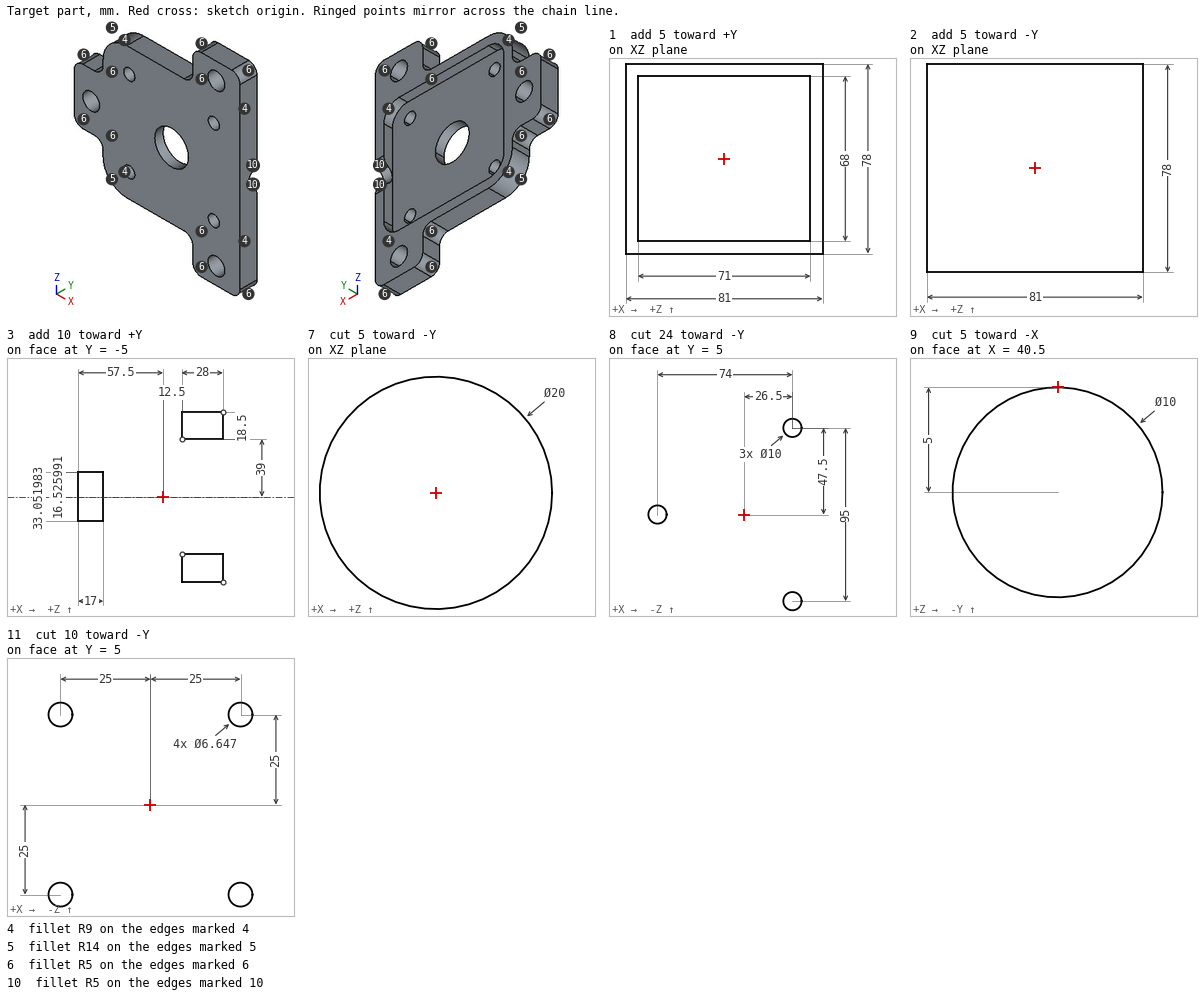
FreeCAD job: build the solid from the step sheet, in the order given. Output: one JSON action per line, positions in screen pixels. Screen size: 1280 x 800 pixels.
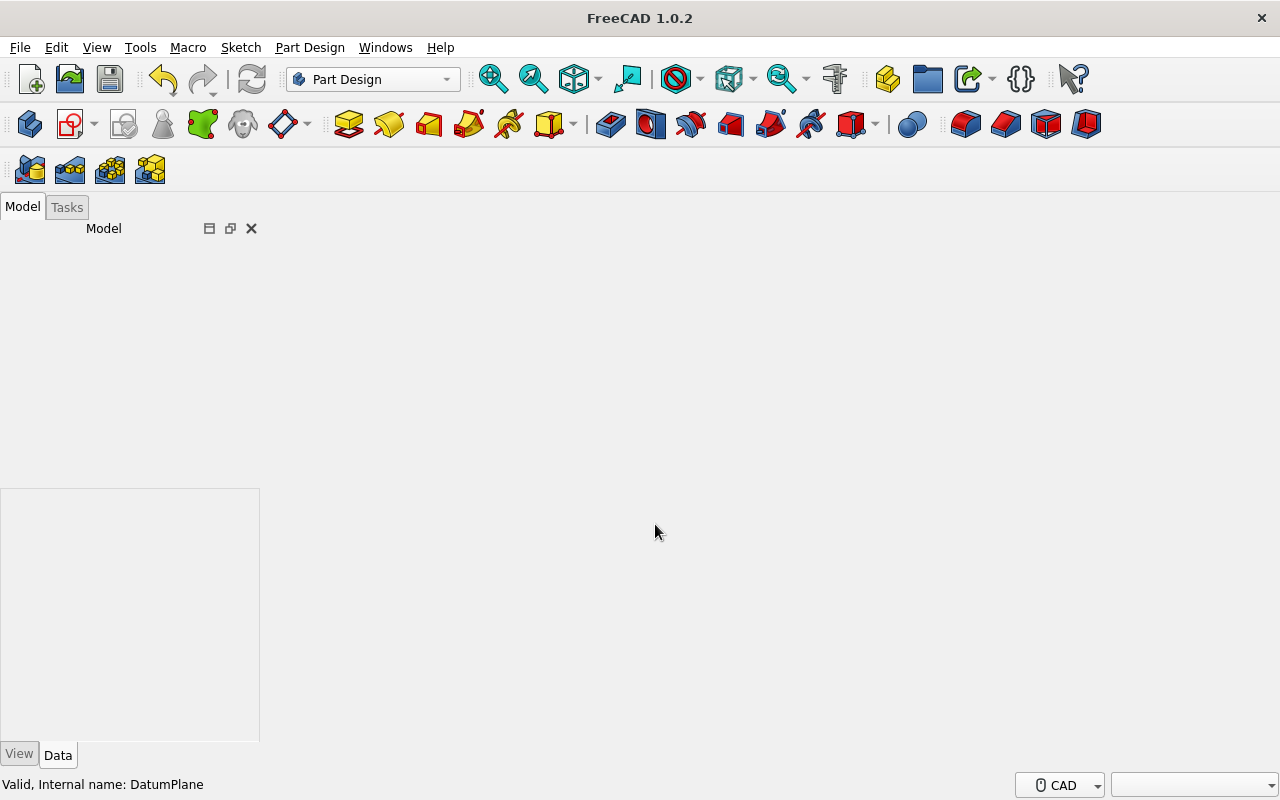
{"action": "left_click", "coordinate": [30, 80]}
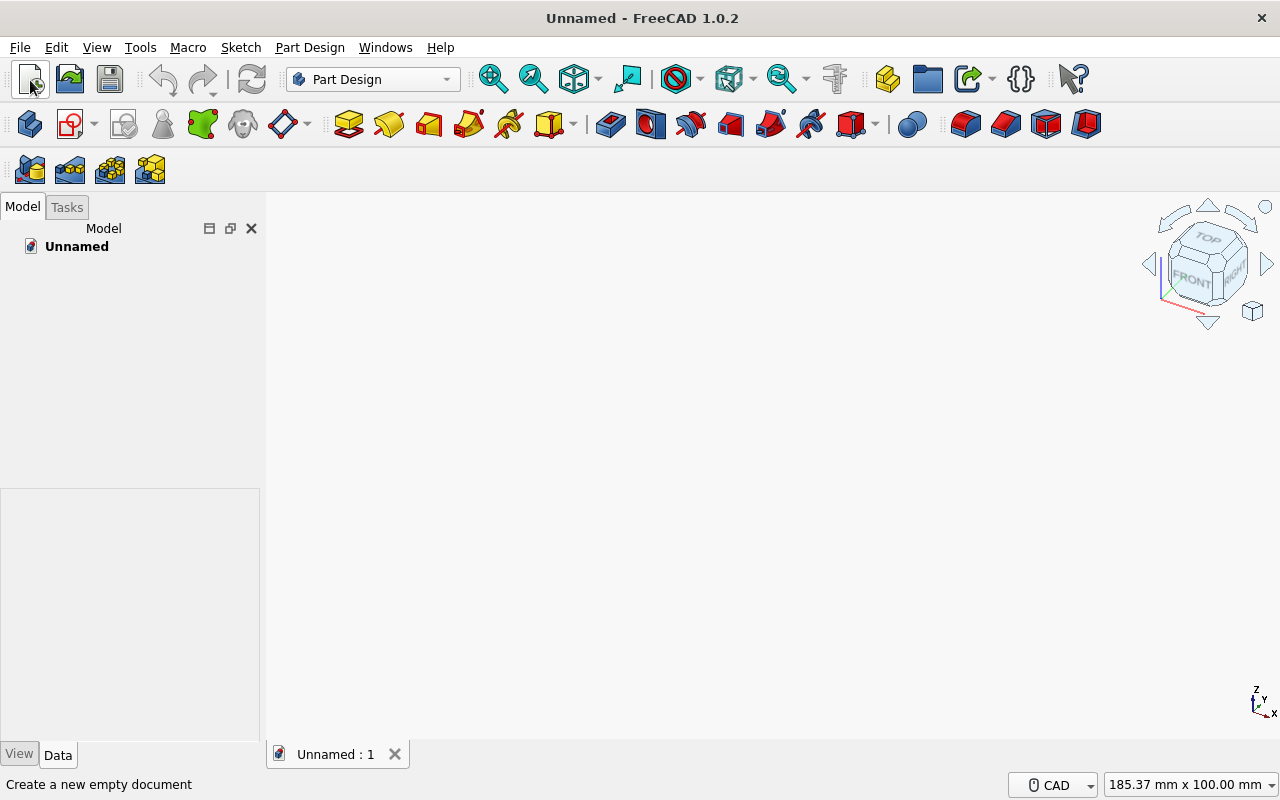
{"action": "left_click", "coordinate": [70, 124]}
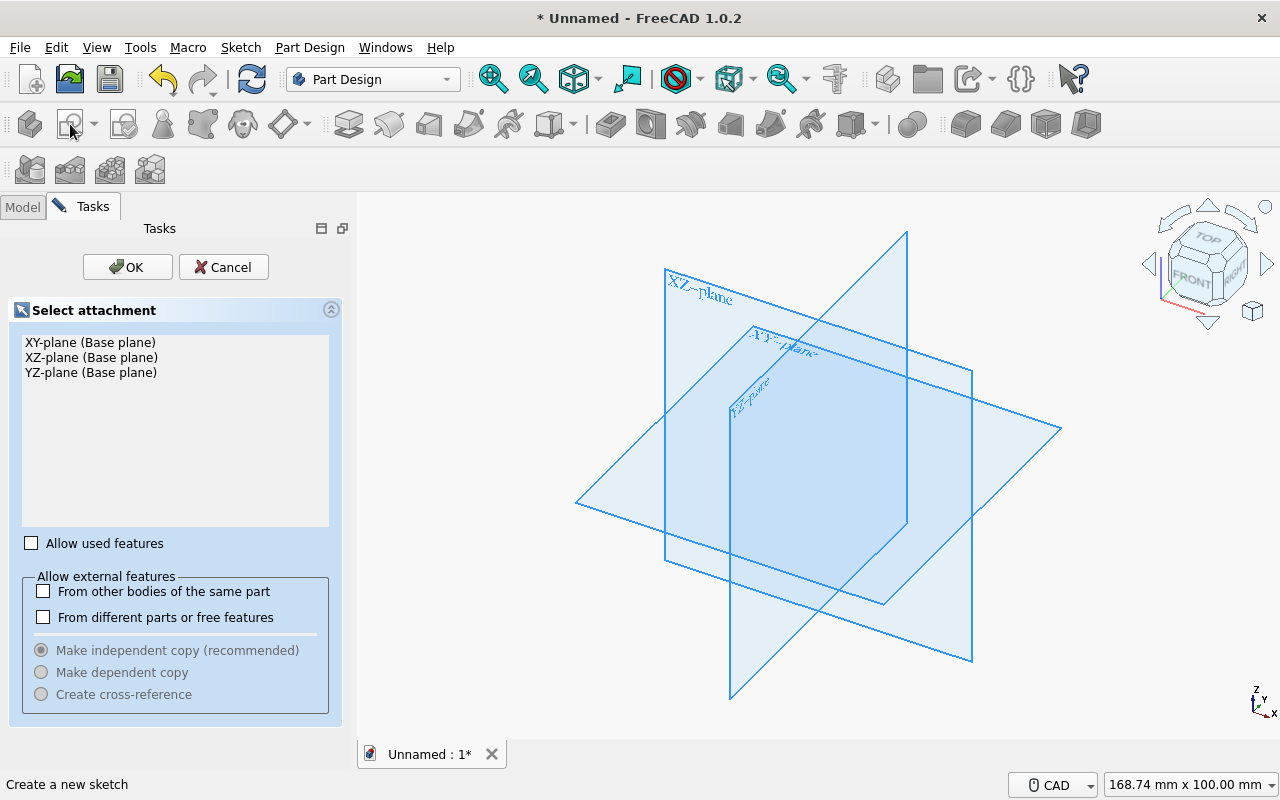
{"action": "left_click", "coordinate": [82, 358]}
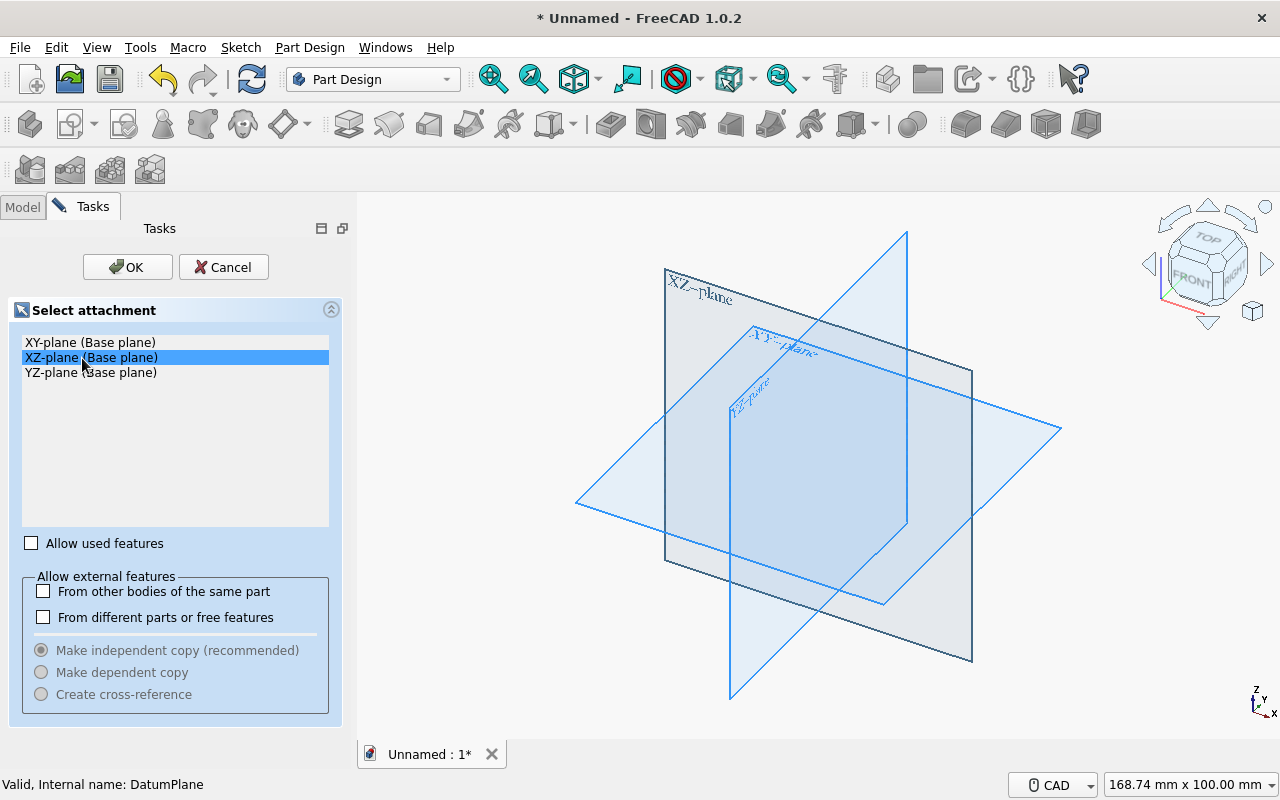
{"action": "left_click", "coordinate": [128, 267]}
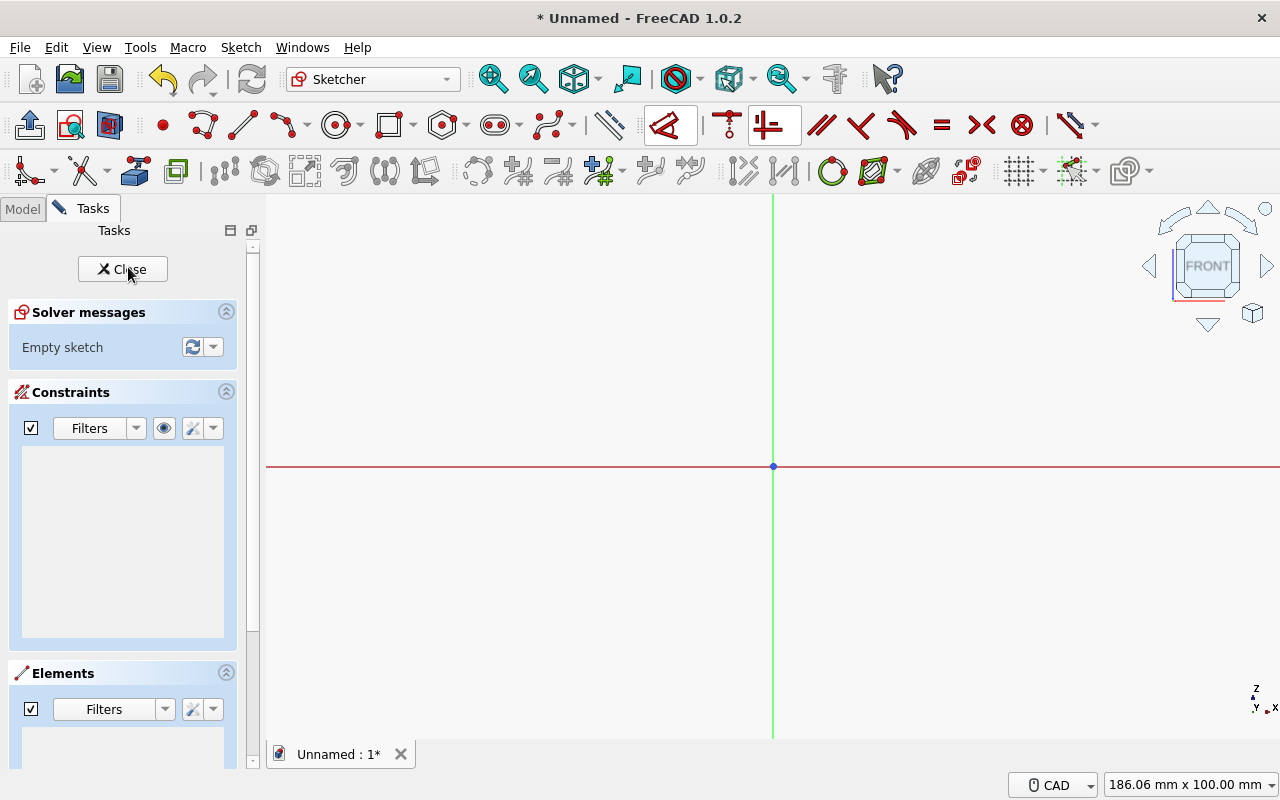
{"action": "key", "text": "g v"}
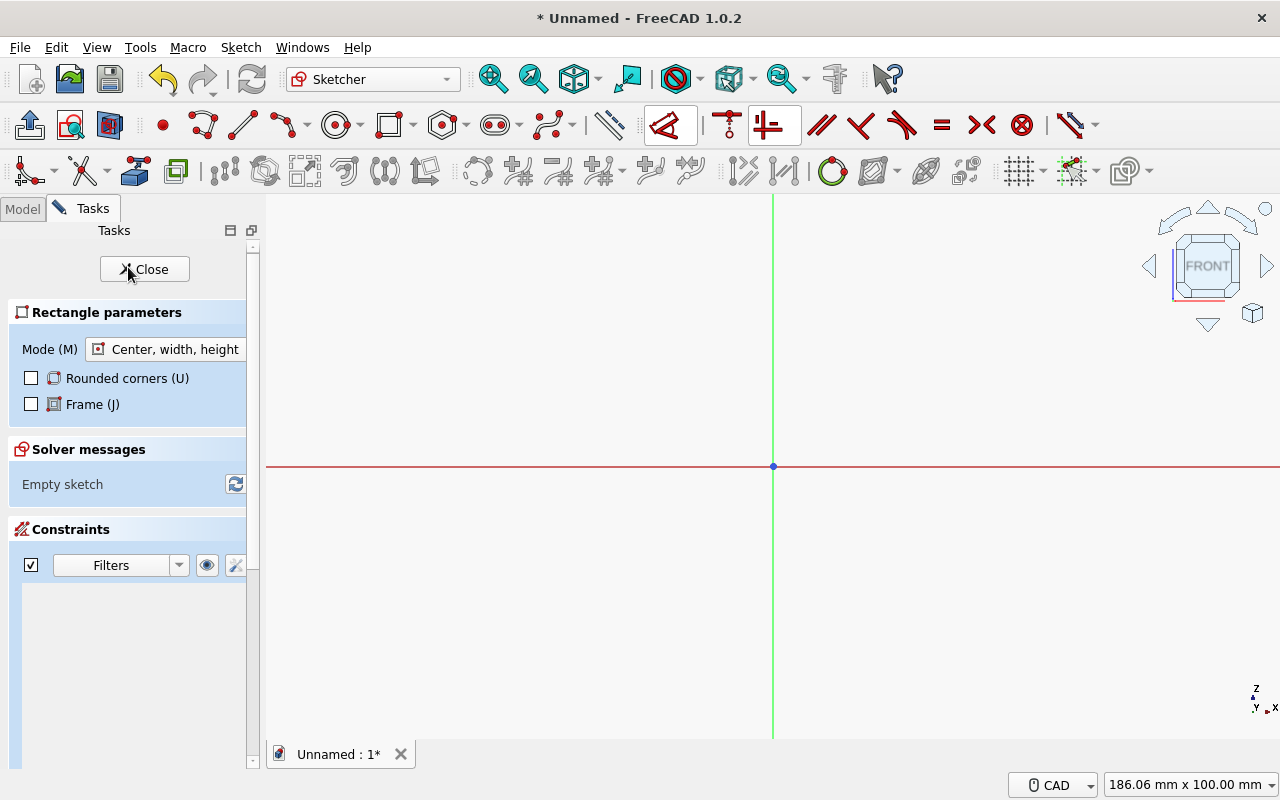
{"action": "left_click", "coordinate": [773, 466]}
{"action": "left_click", "coordinate": [994, 254]}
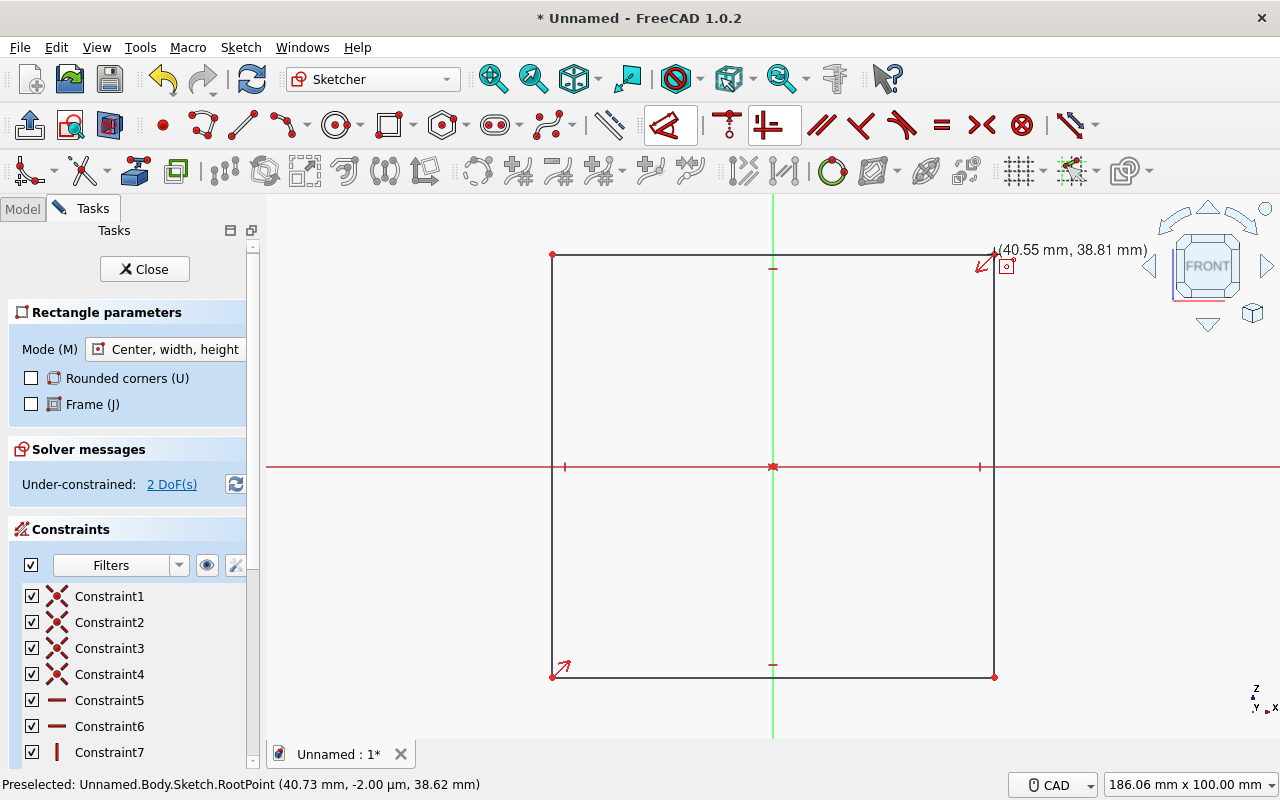
{"action": "left_click", "coordinate": [773, 466]}
{"action": "left_click", "coordinate": [966, 281]}
{"action": "key", "text": "Escape"}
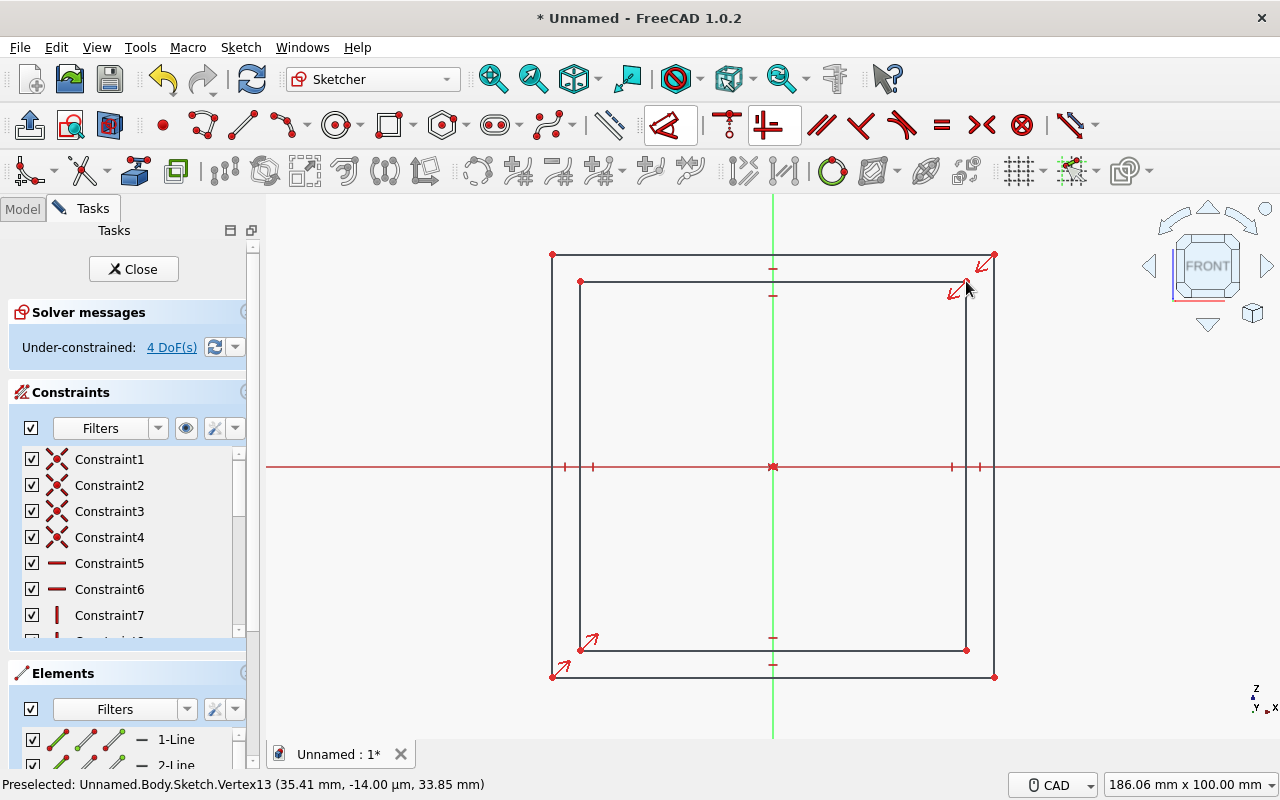
{"action": "left_click", "coordinate": [664, 126]}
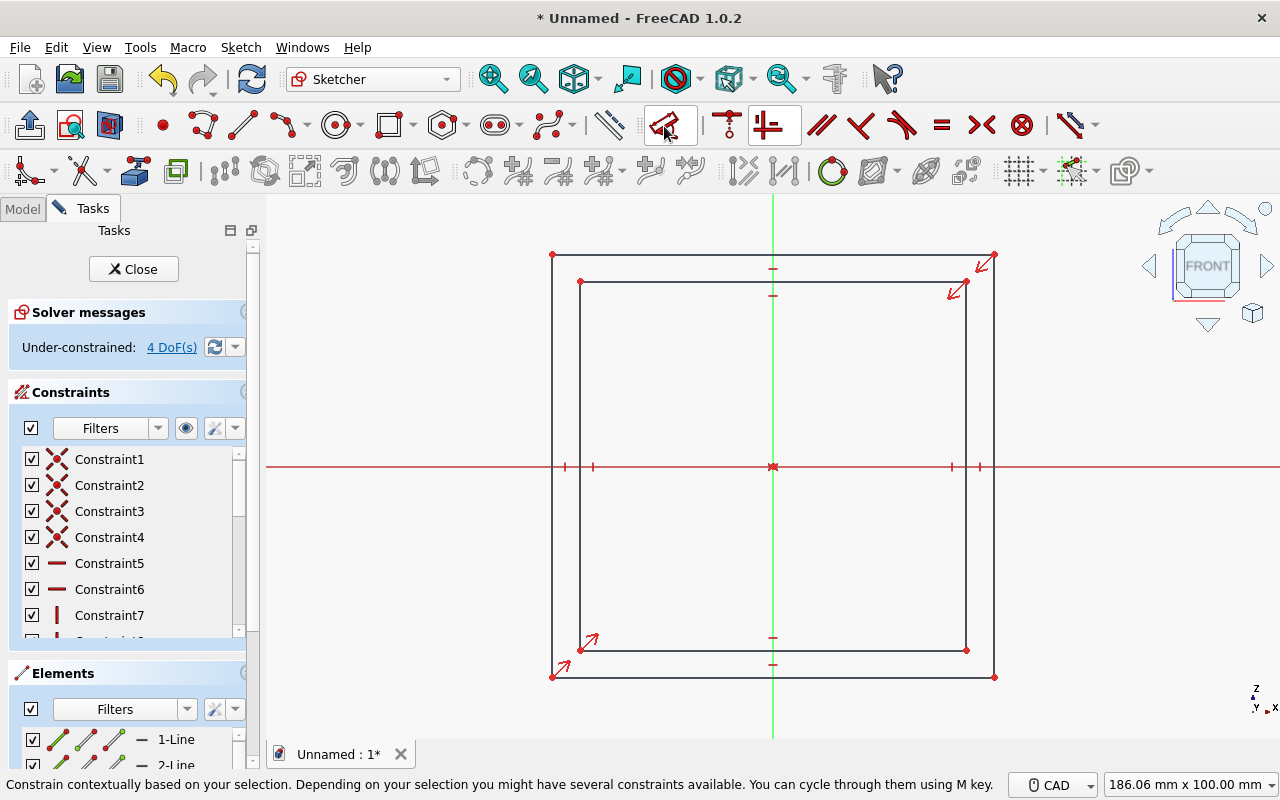
{"action": "left_click", "coordinate": [685, 678]}
{"action": "left_click", "coordinate": [671, 620]}